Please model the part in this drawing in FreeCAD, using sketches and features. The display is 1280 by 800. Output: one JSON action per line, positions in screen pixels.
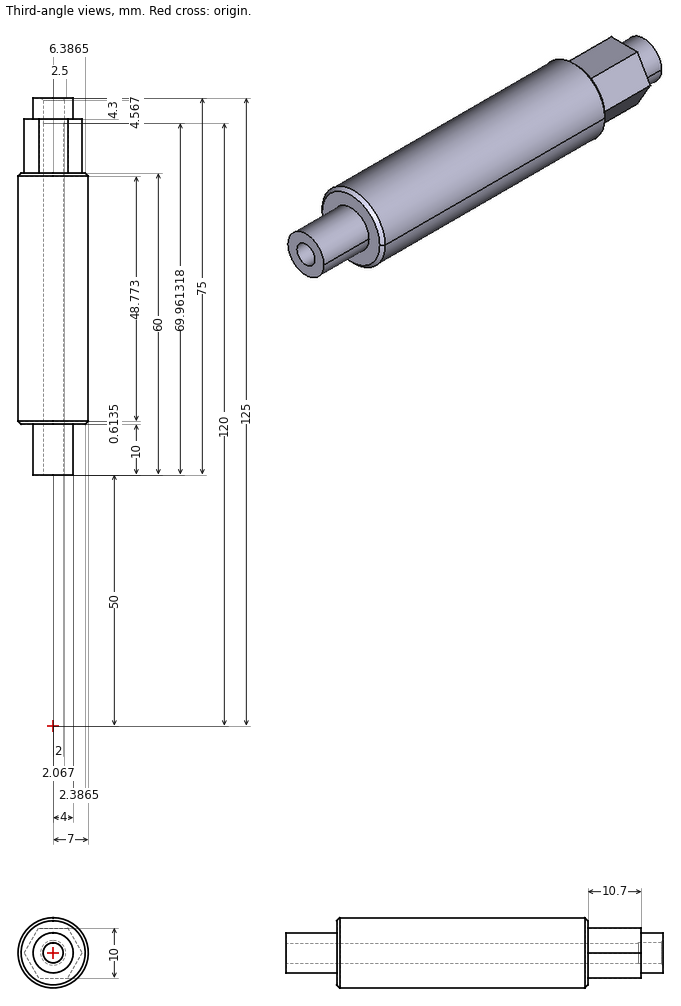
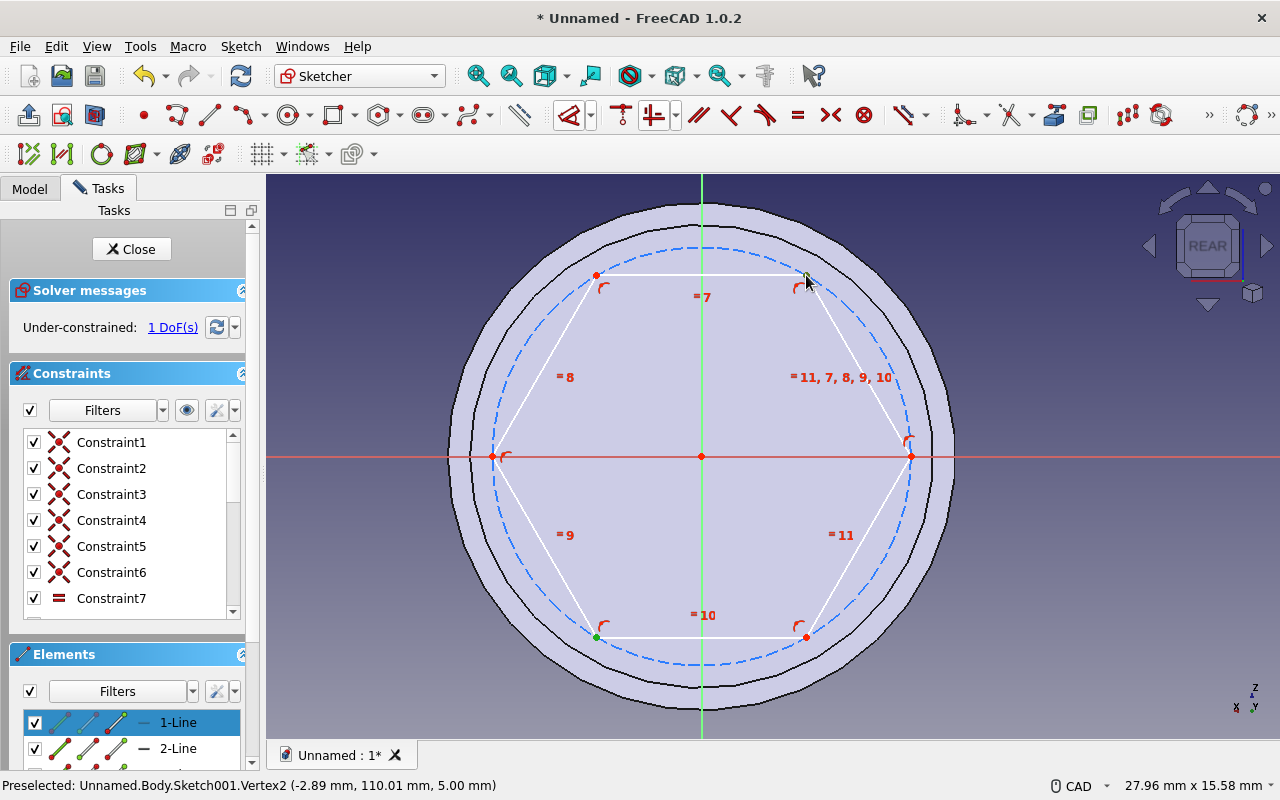
{"action": "key", "text": "i"}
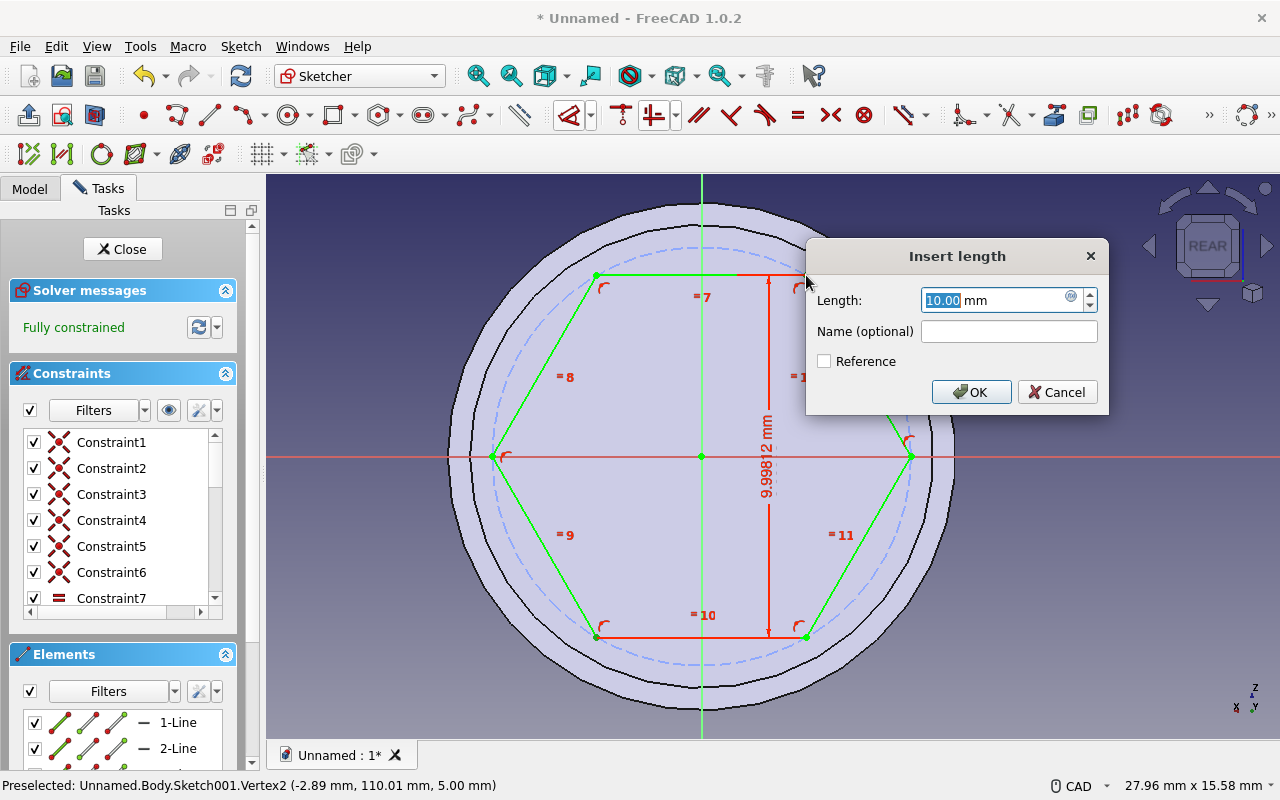
{"action": "type", "text": "10"}
{"action": "key", "text": "Return"}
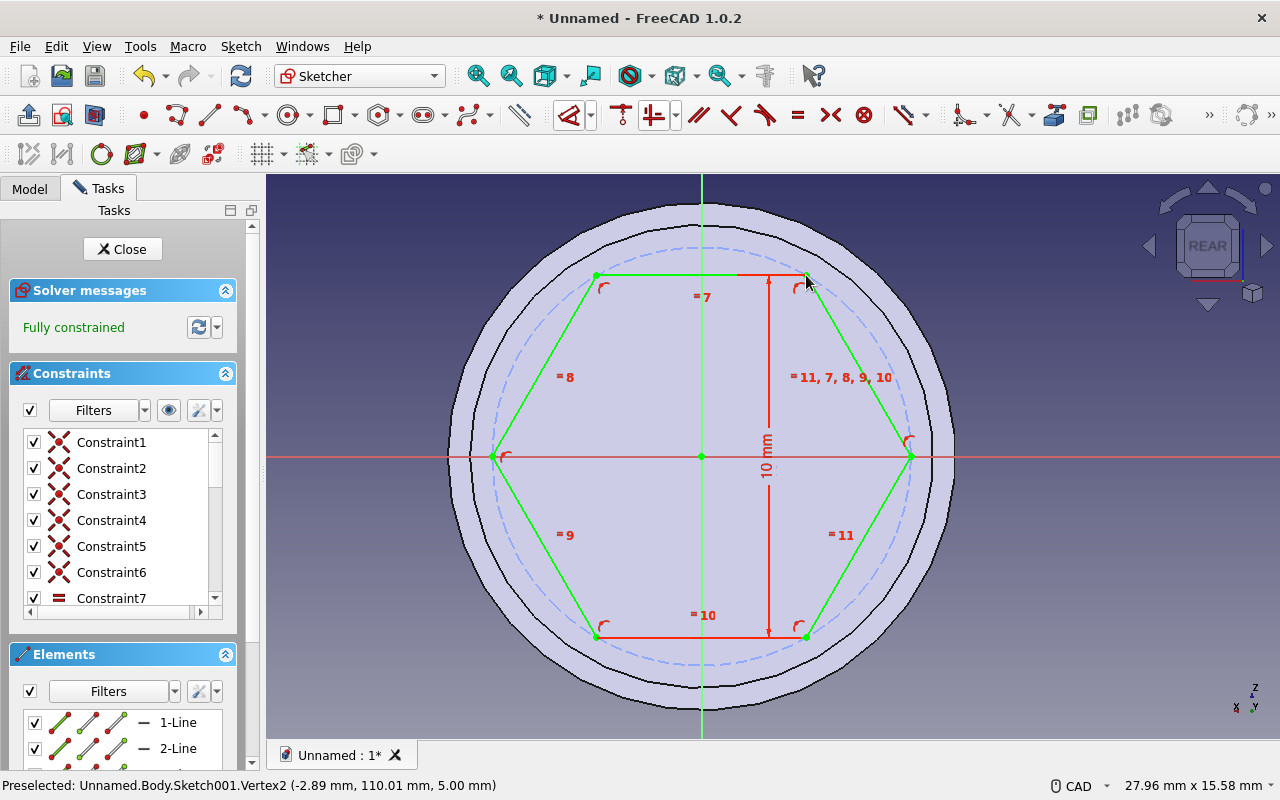
{"action": "left_click", "coordinate": [123, 249]}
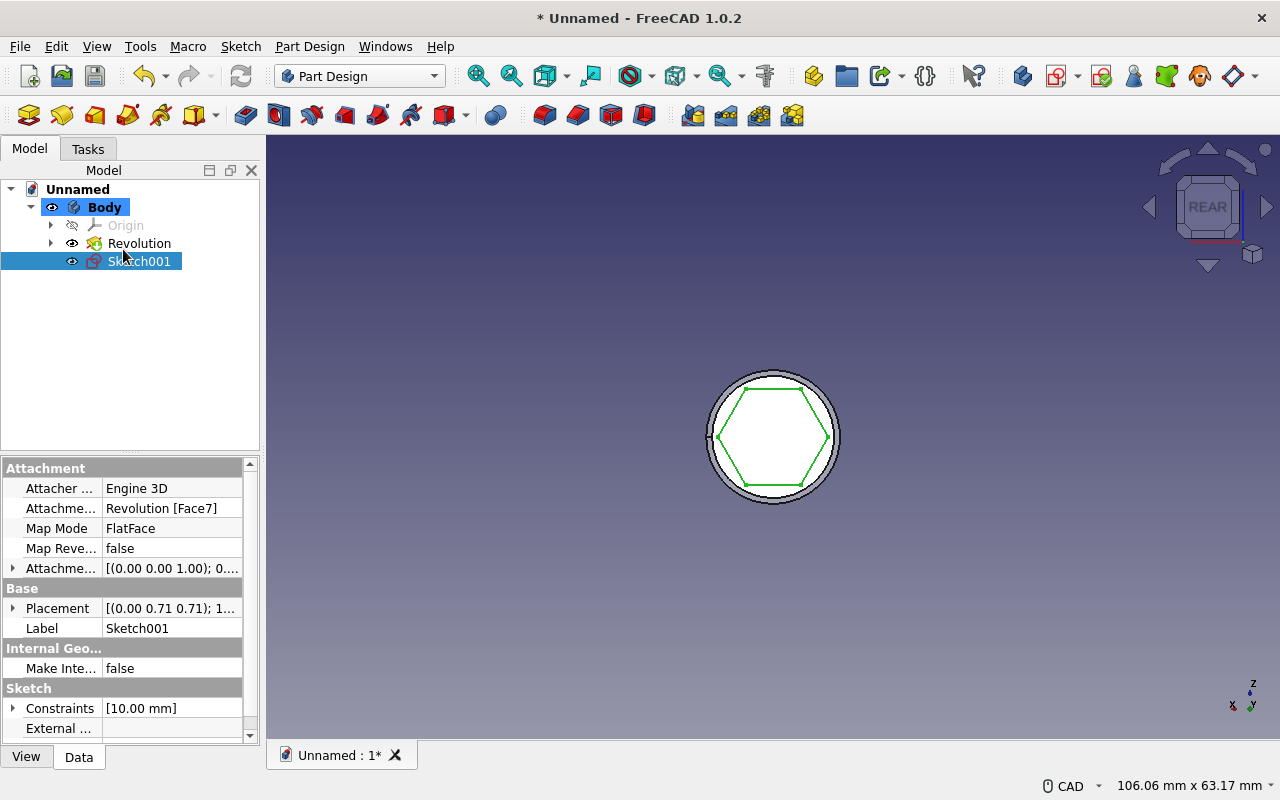
{"action": "left_click", "coordinate": [29, 116]}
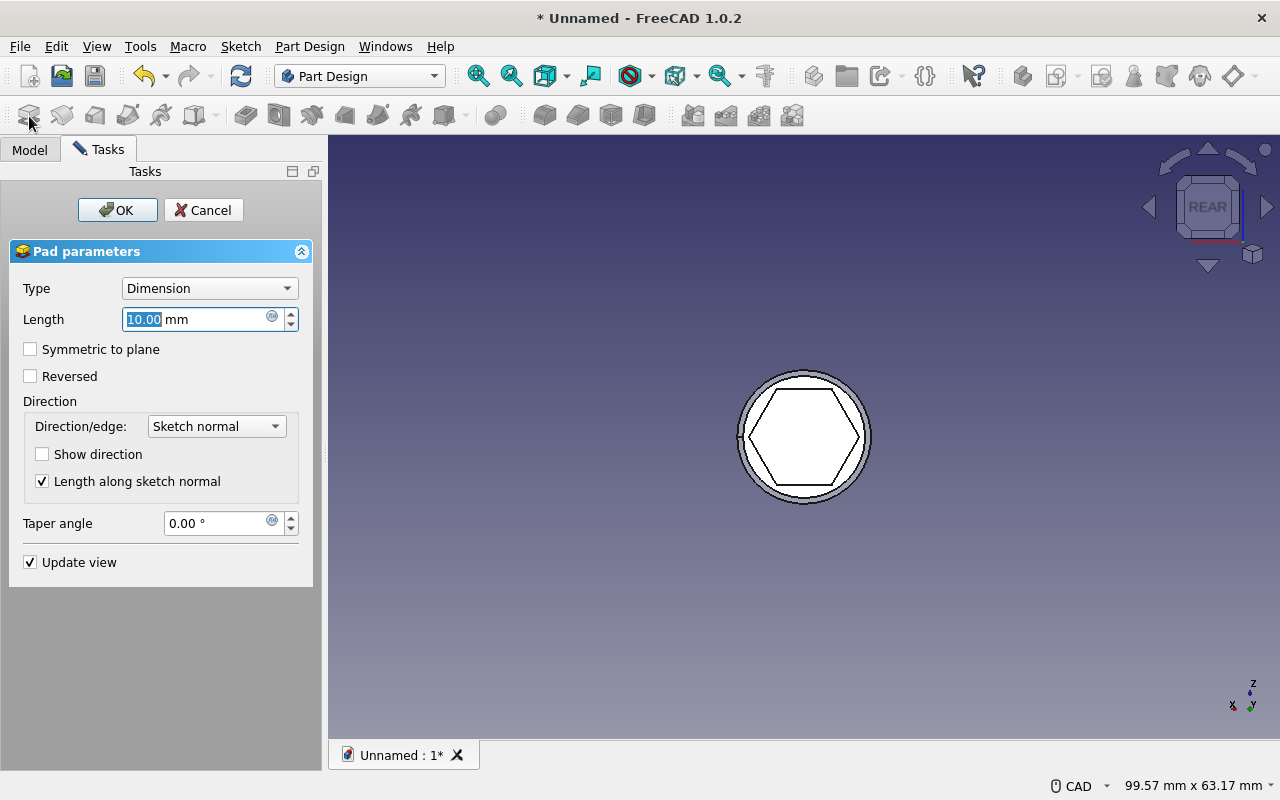
{"action": "type", "text": "10.7"}
{"action": "key", "text": "Tab"}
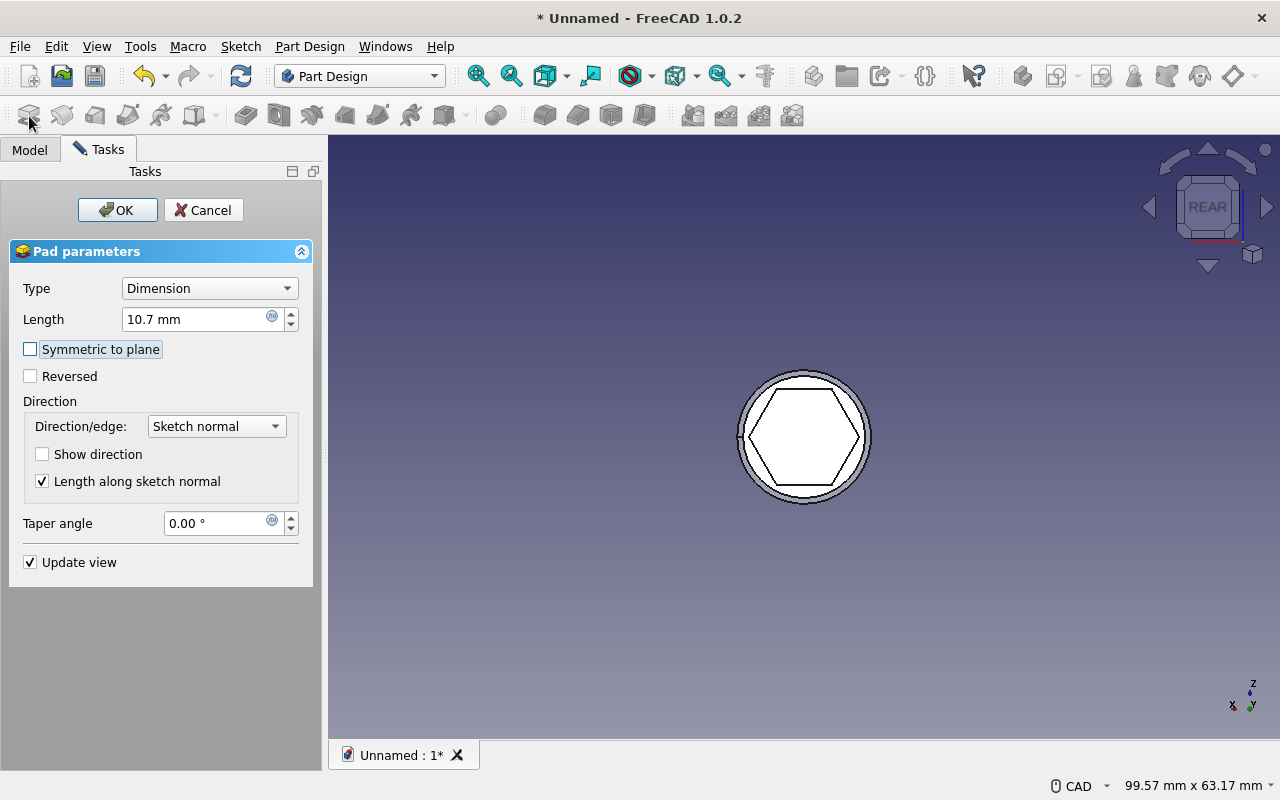
{"action": "left_click", "coordinate": [118, 210]}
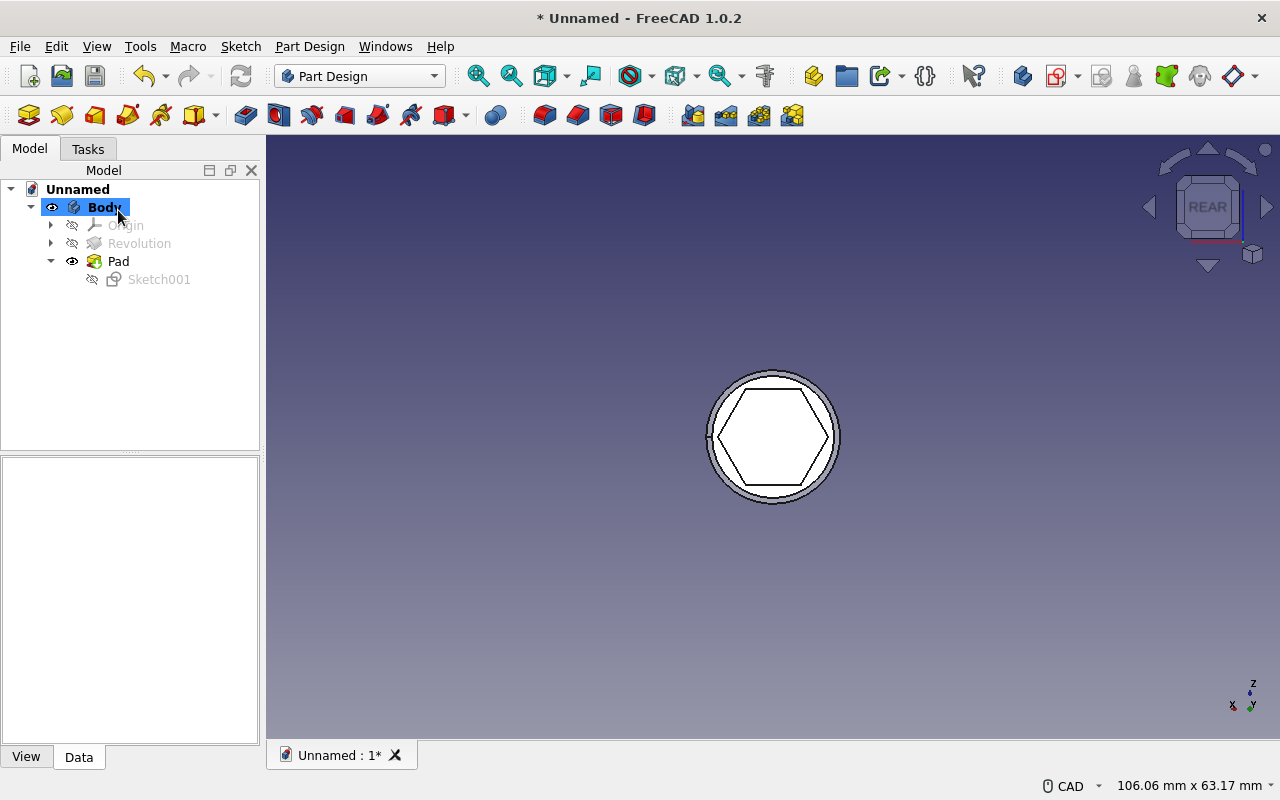
{"action": "key", "text": "v f"}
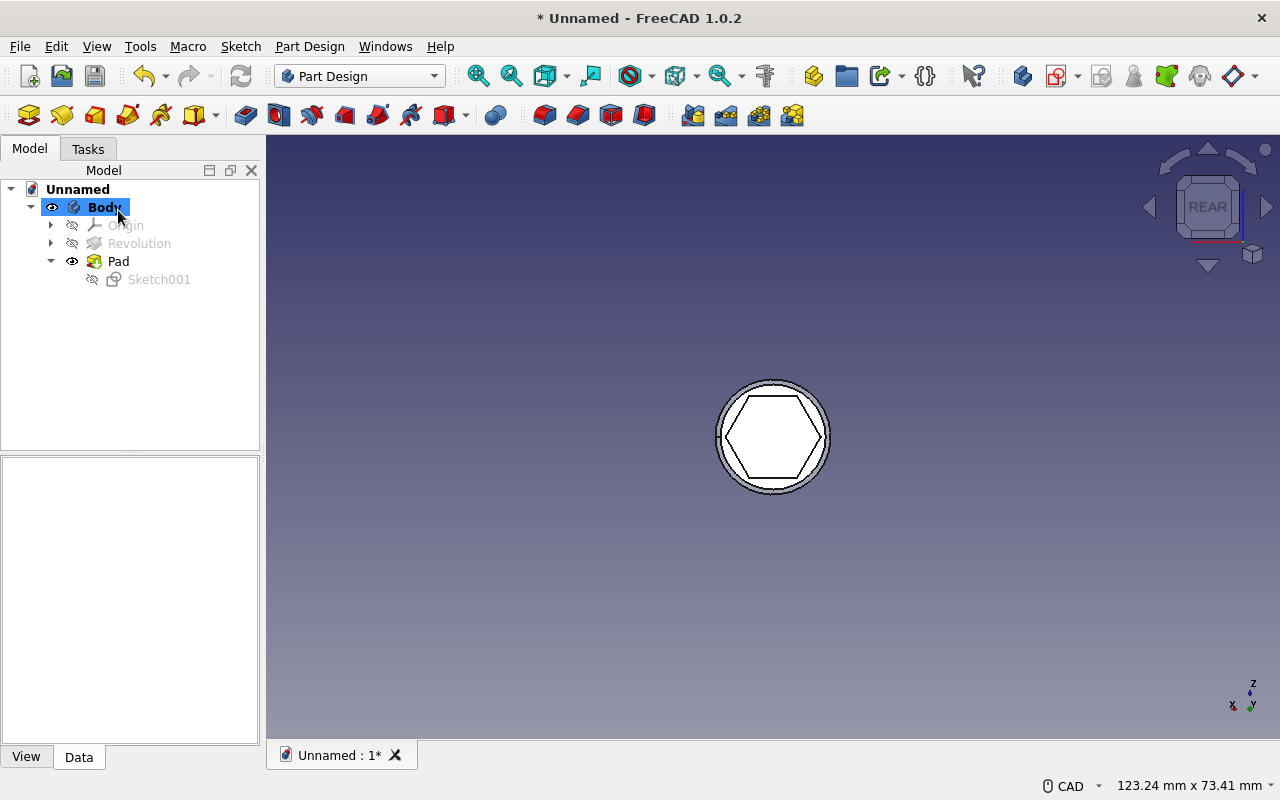
{"action": "left_click", "coordinate": [1056, 76]}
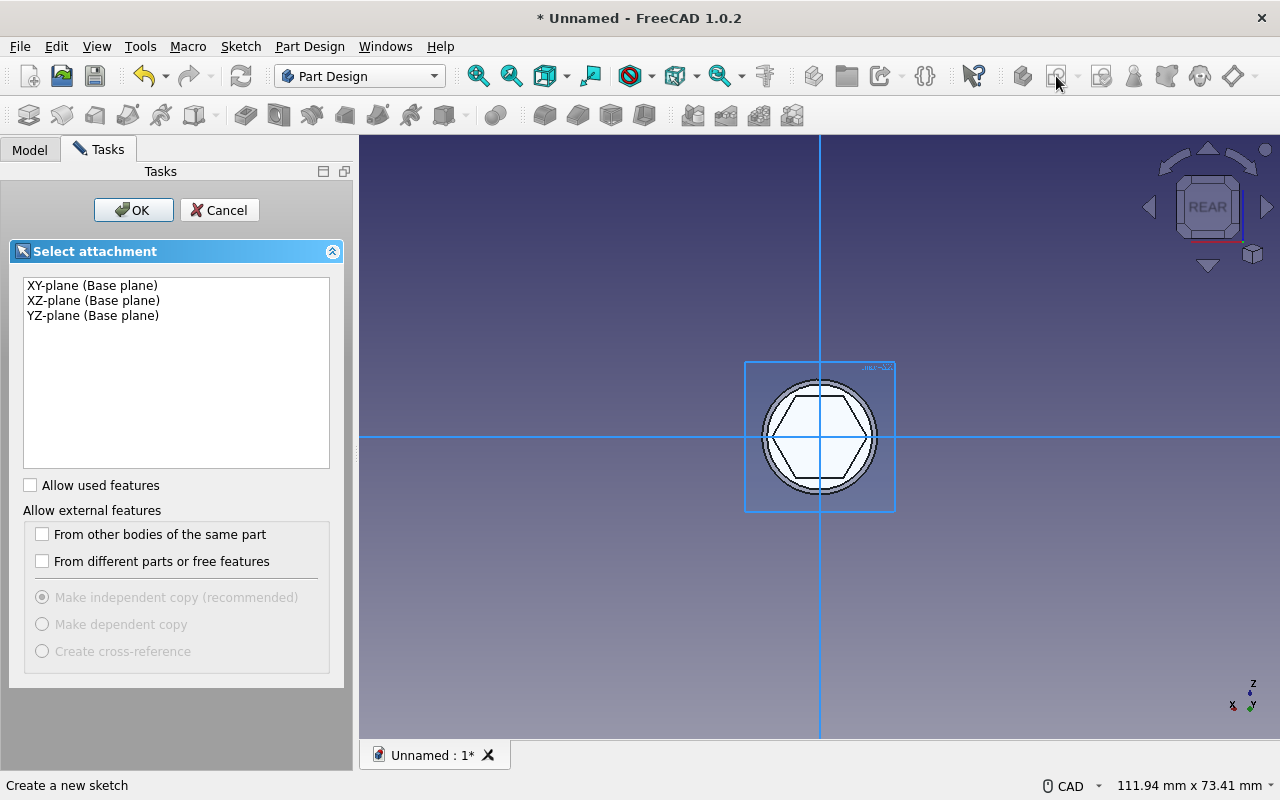
{"action": "left_click", "coordinate": [84, 286]}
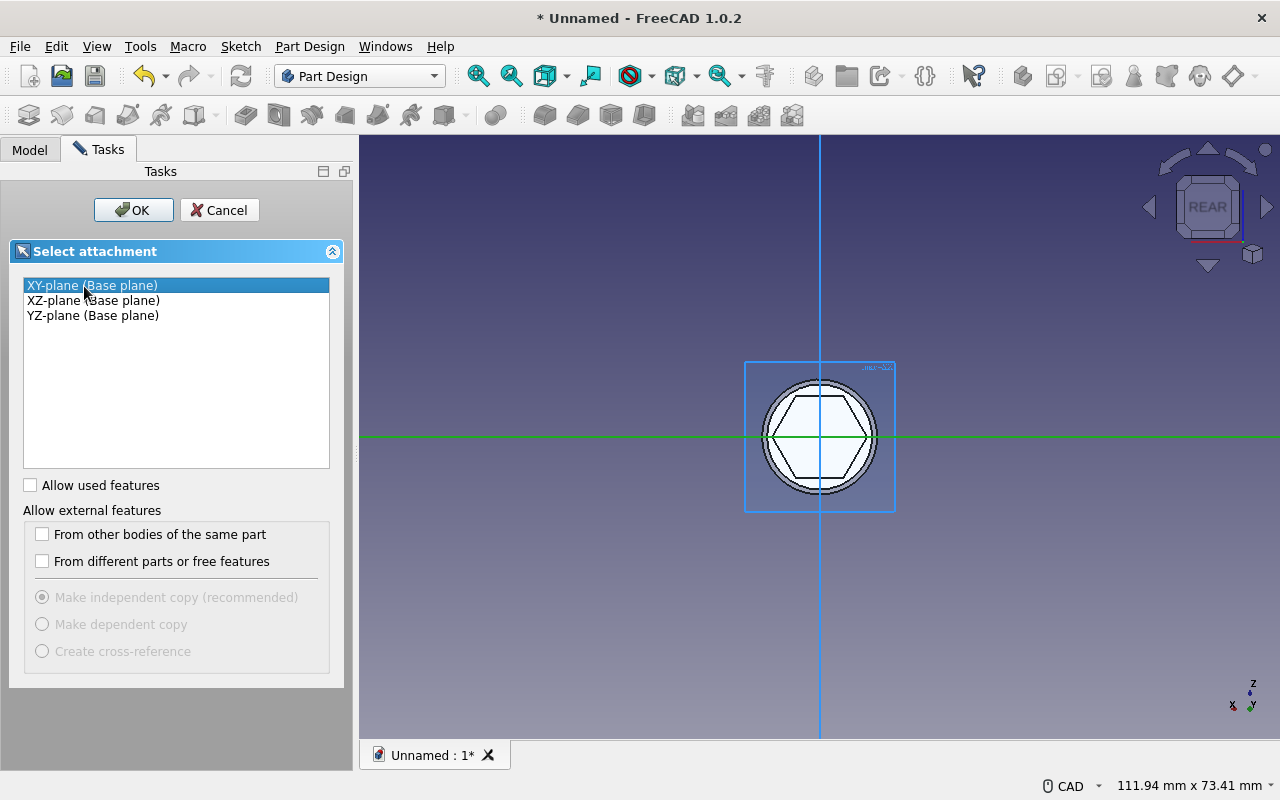
{"action": "left_click", "coordinate": [134, 210]}